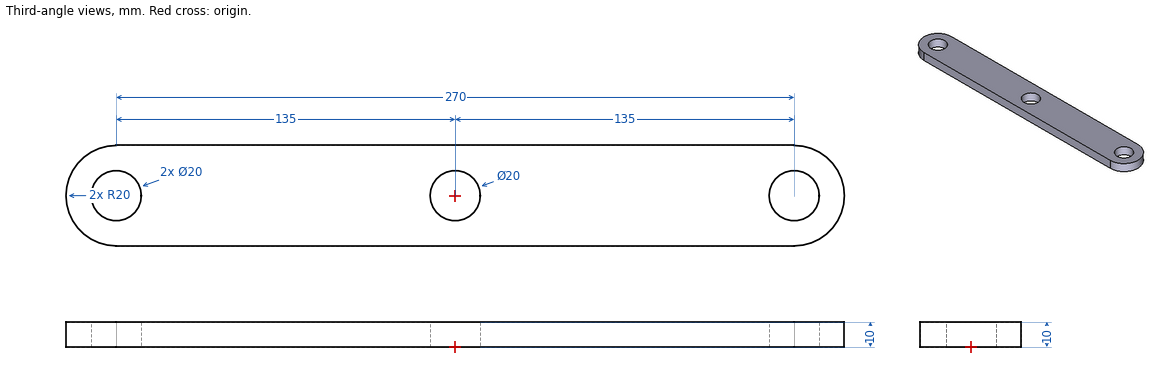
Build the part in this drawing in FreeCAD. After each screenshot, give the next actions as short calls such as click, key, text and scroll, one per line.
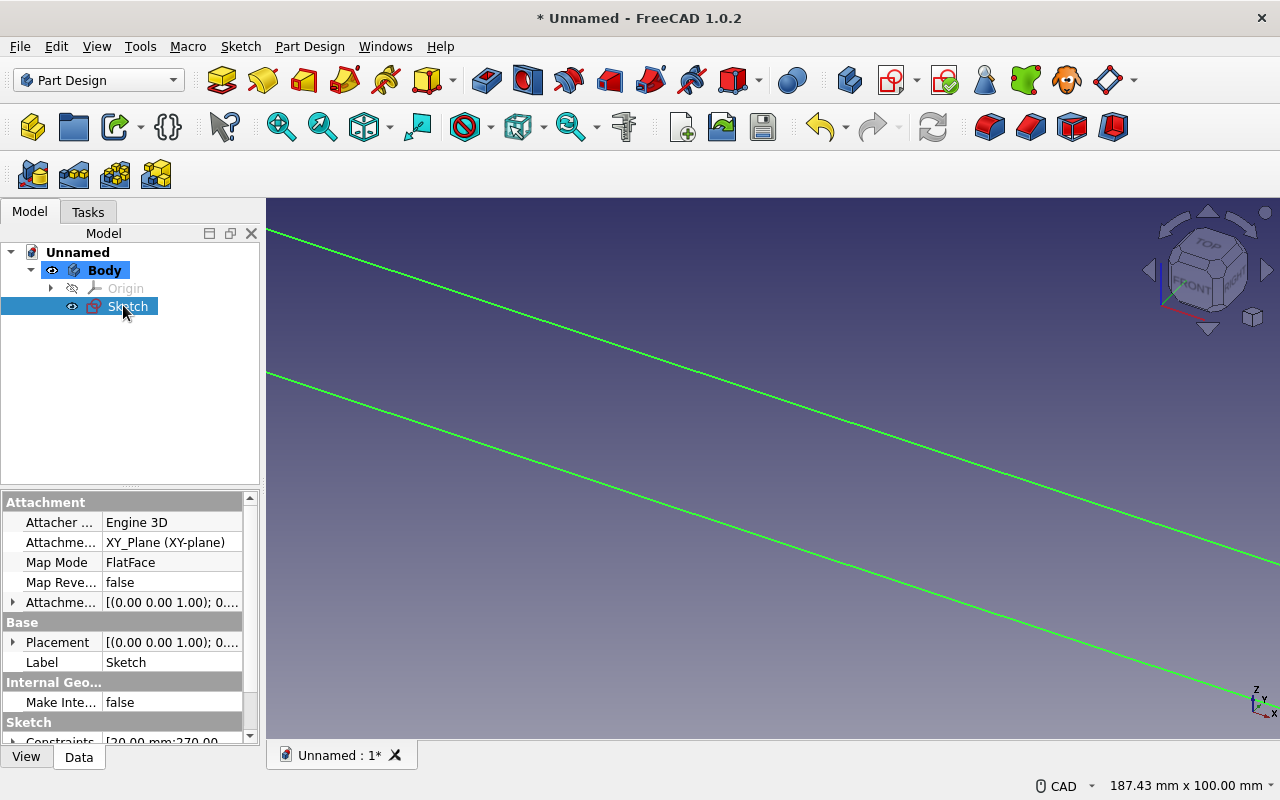
click(222, 80)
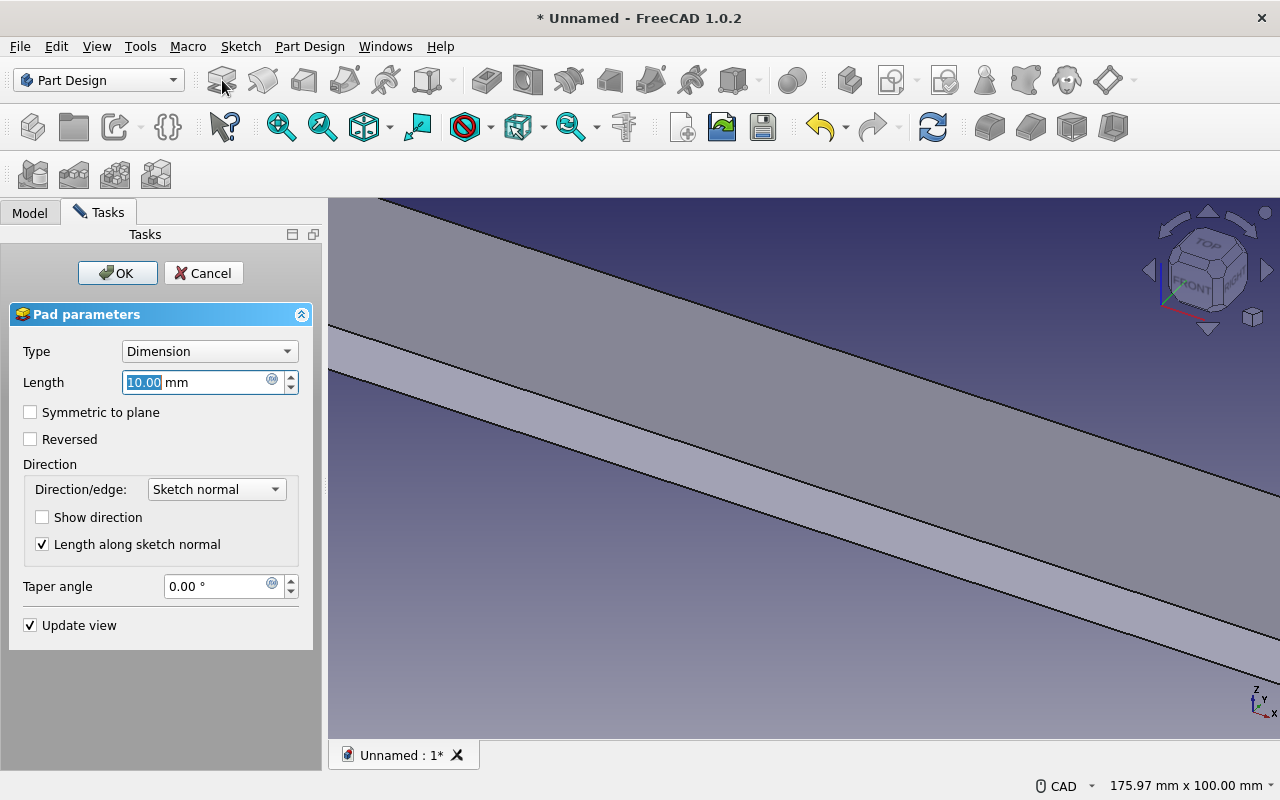
text(10)
key(Tab)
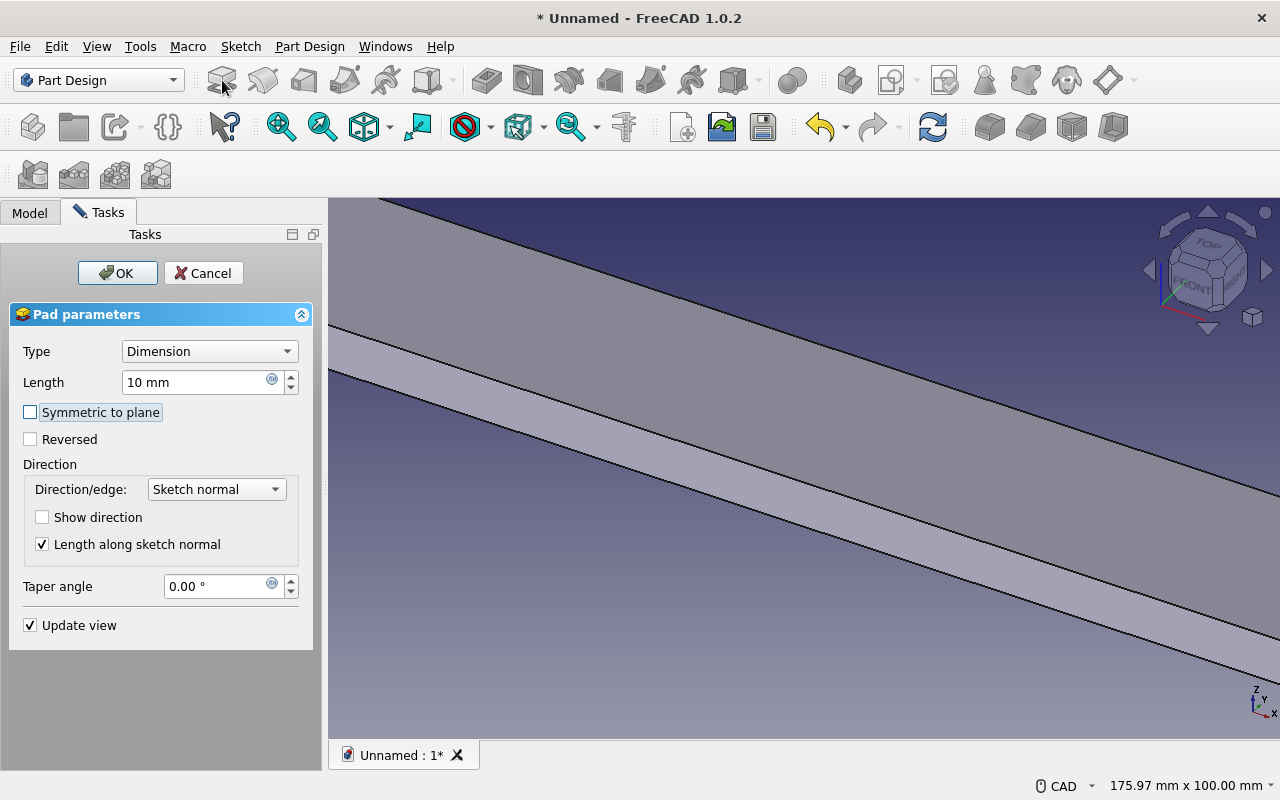
click(118, 273)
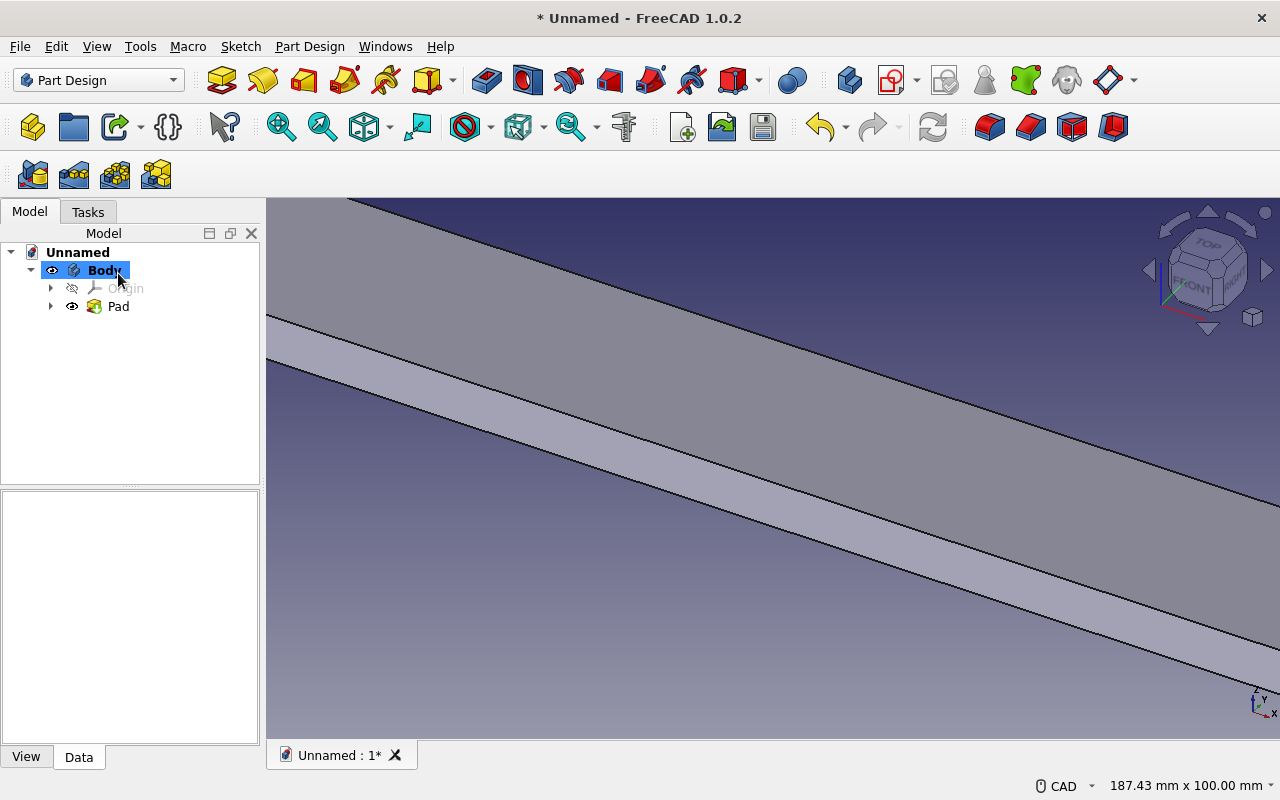
click(282, 128)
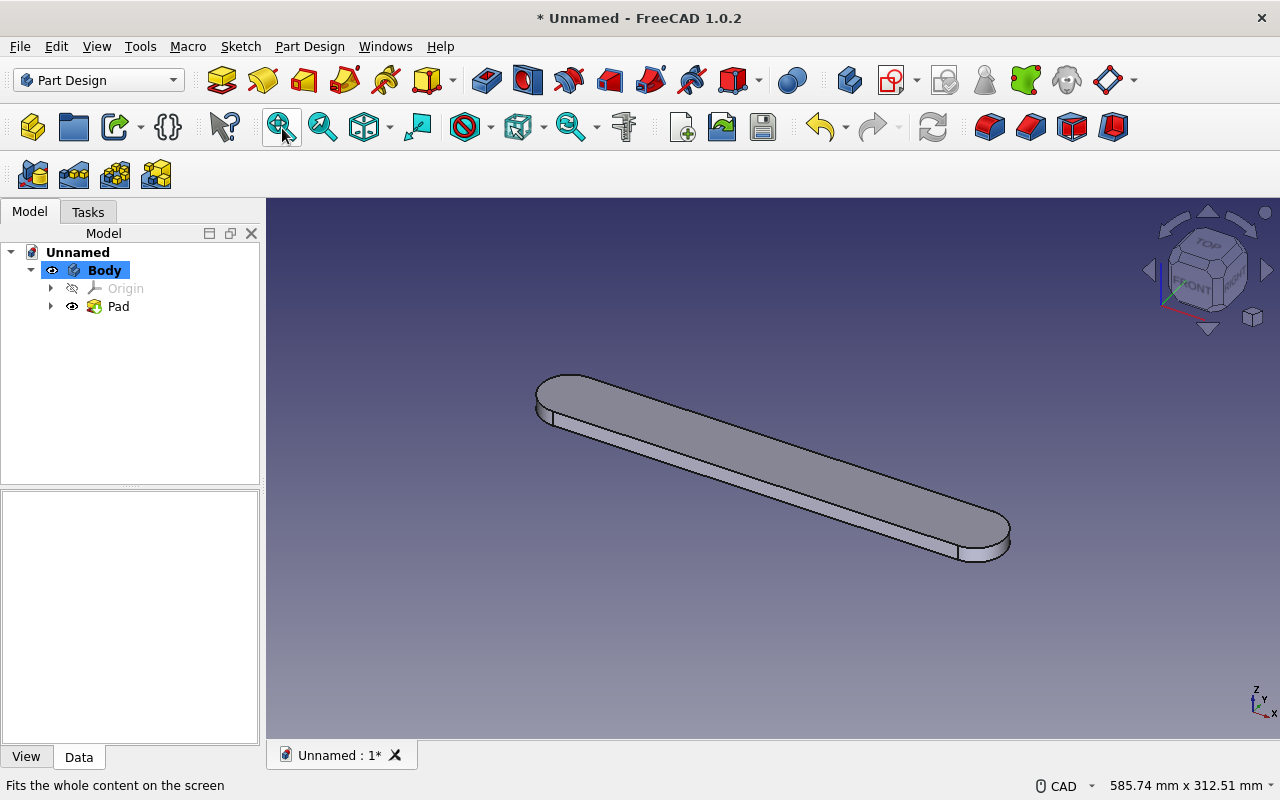
click(972, 526)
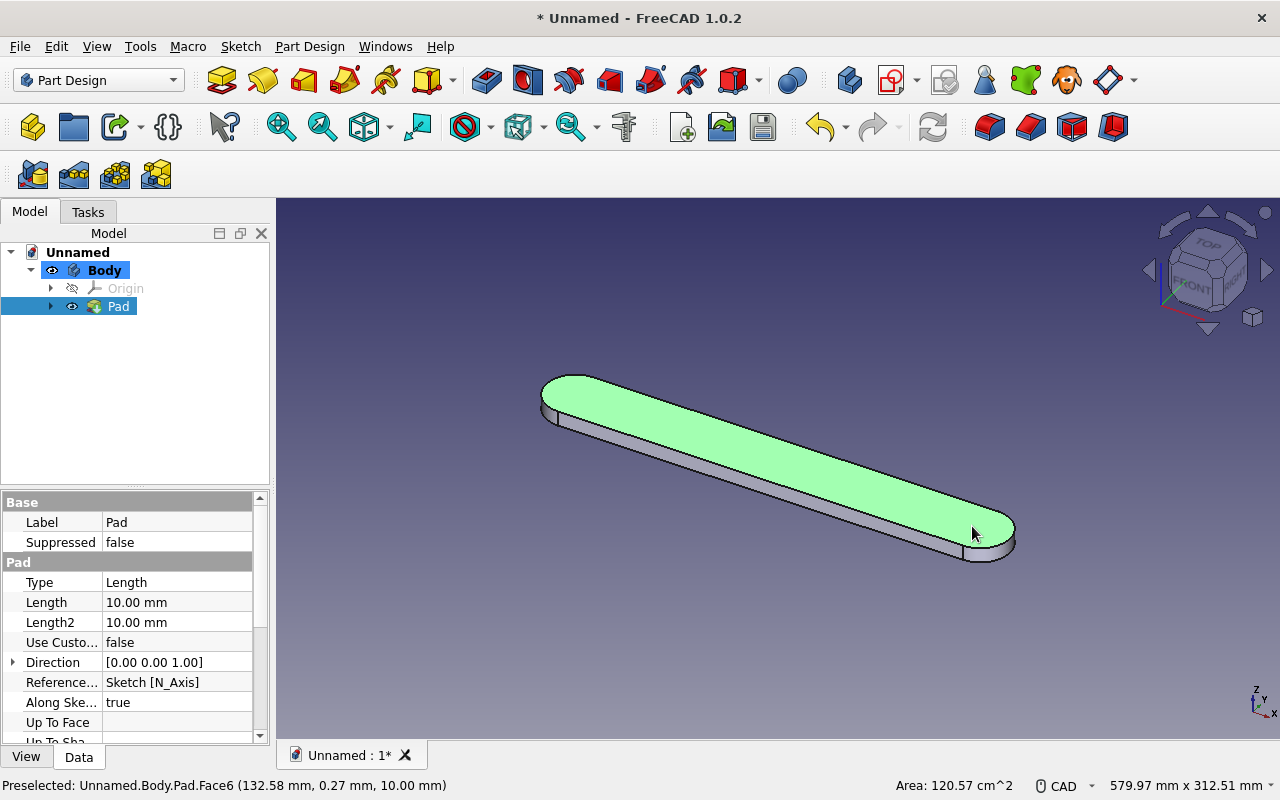
click(890, 80)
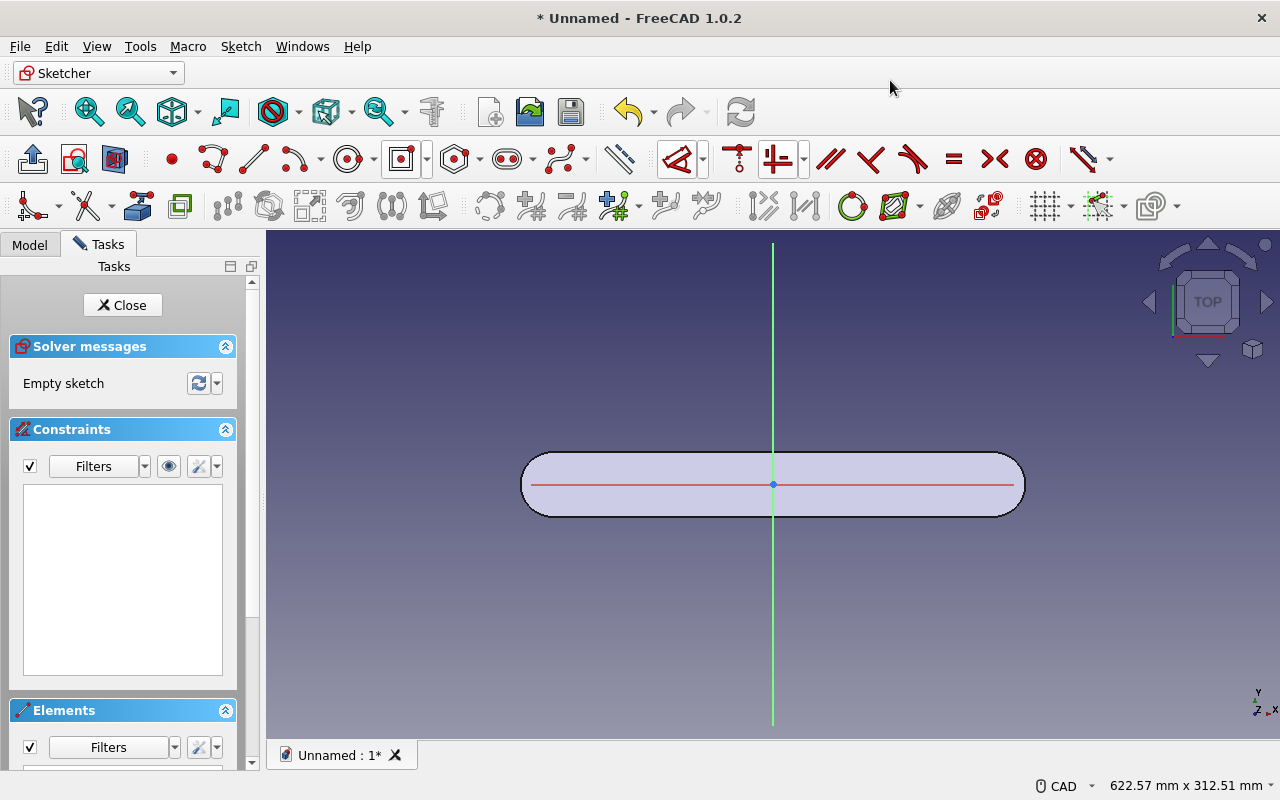
click(348, 160)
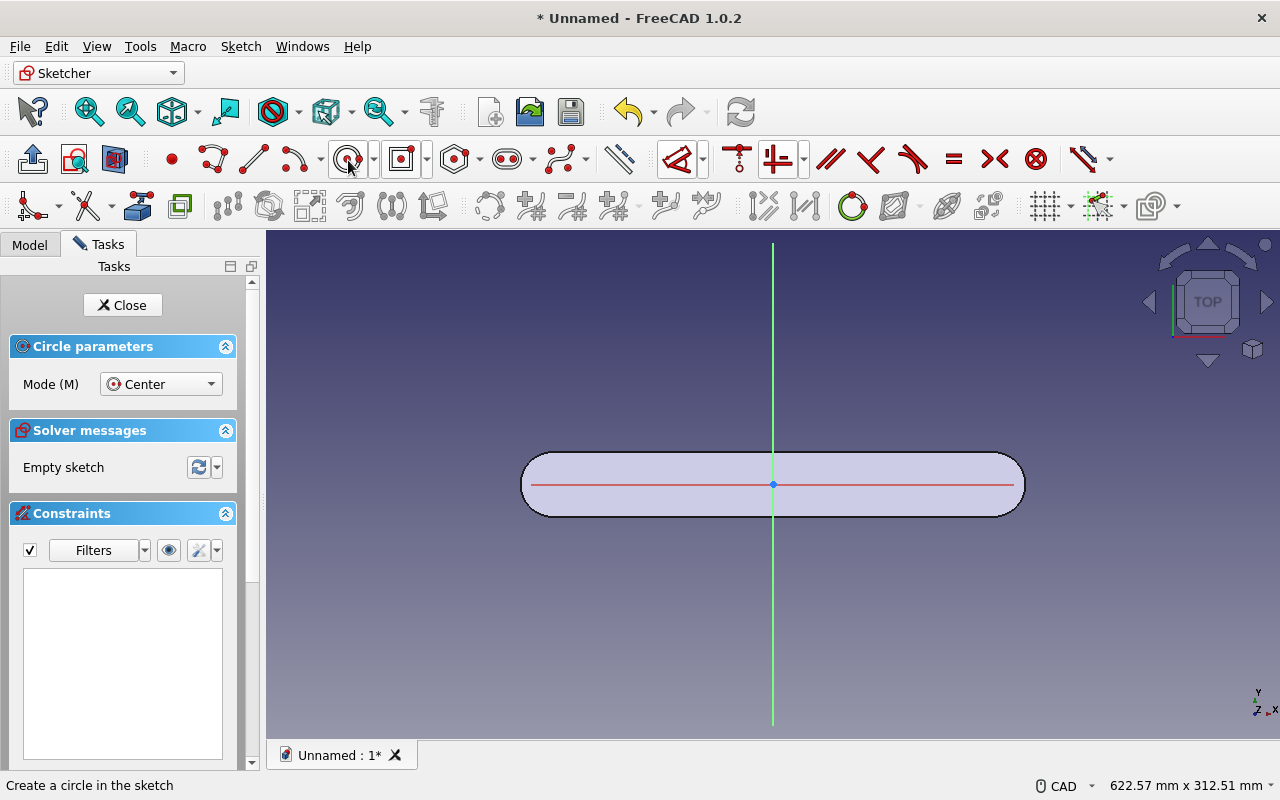
scroll(553, 484, up, 2)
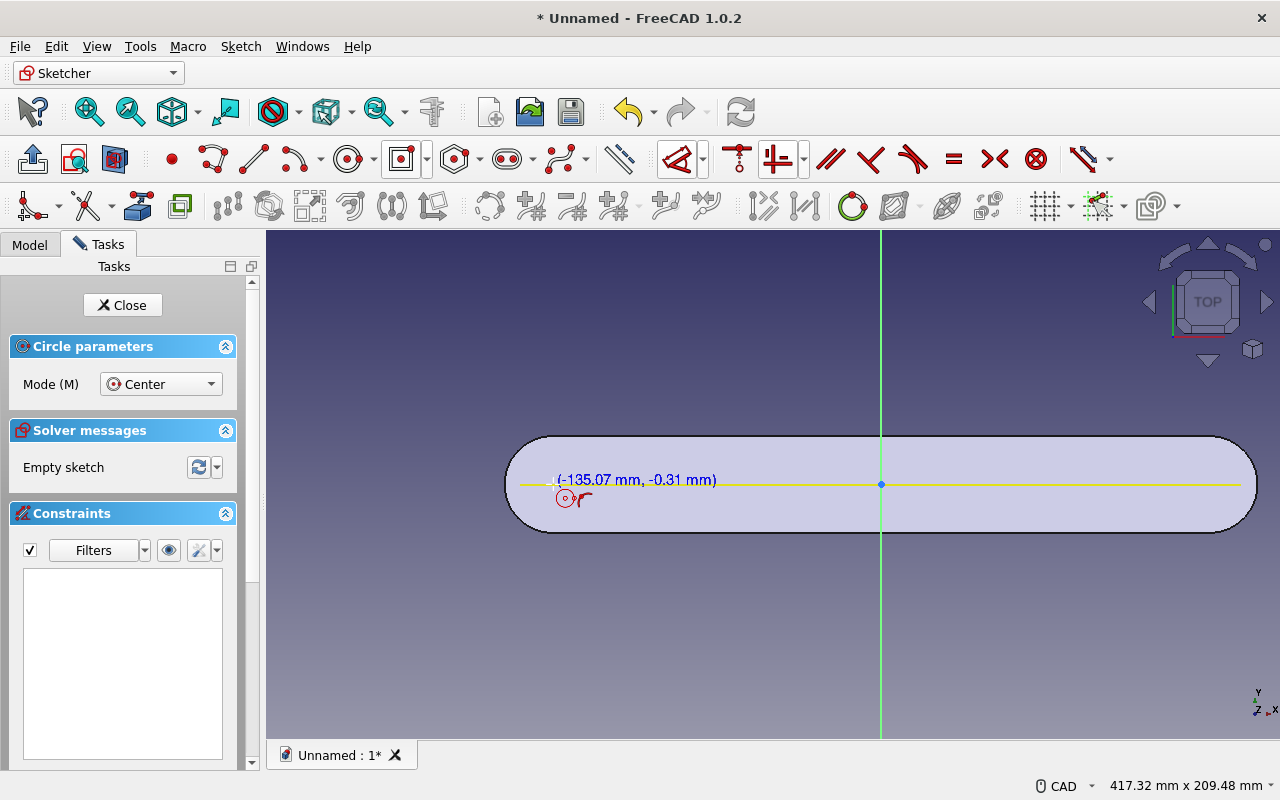
click(553, 484)
click(570, 467)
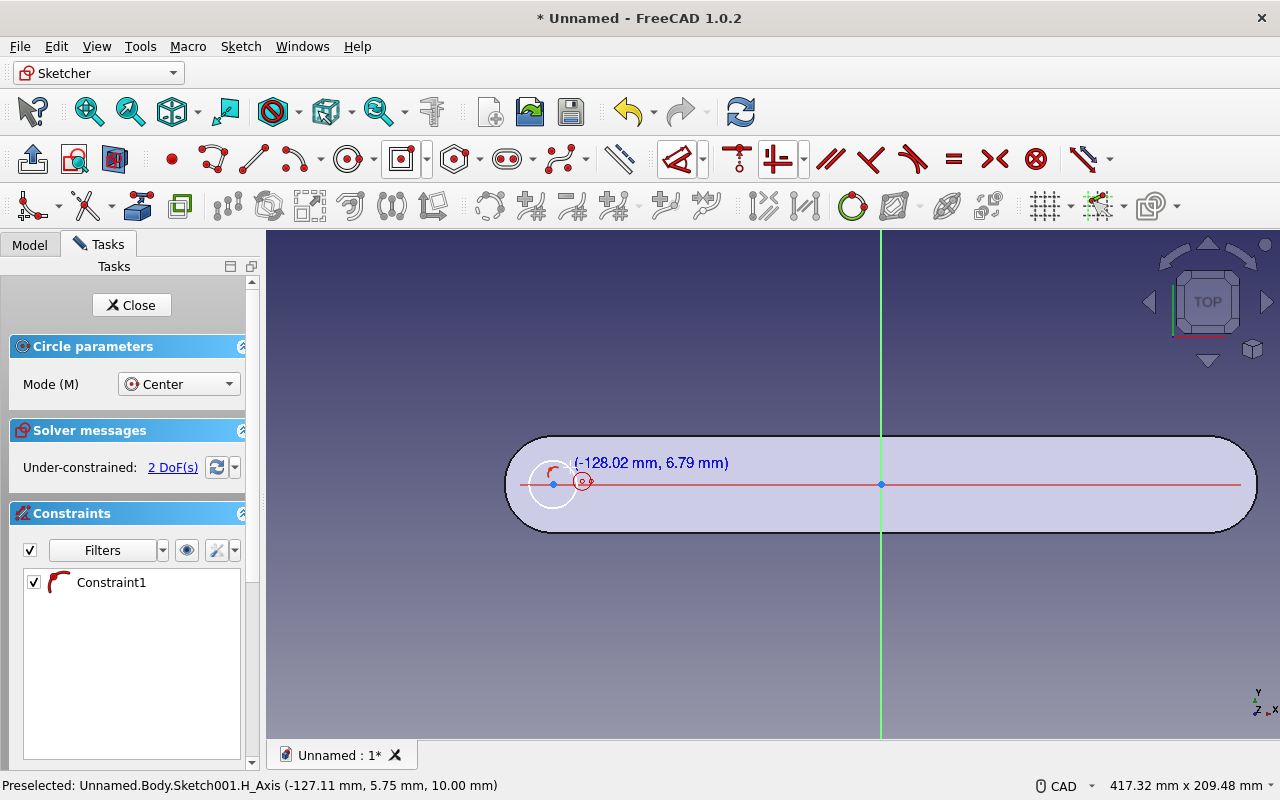
scroll(294, 485, down, 1)